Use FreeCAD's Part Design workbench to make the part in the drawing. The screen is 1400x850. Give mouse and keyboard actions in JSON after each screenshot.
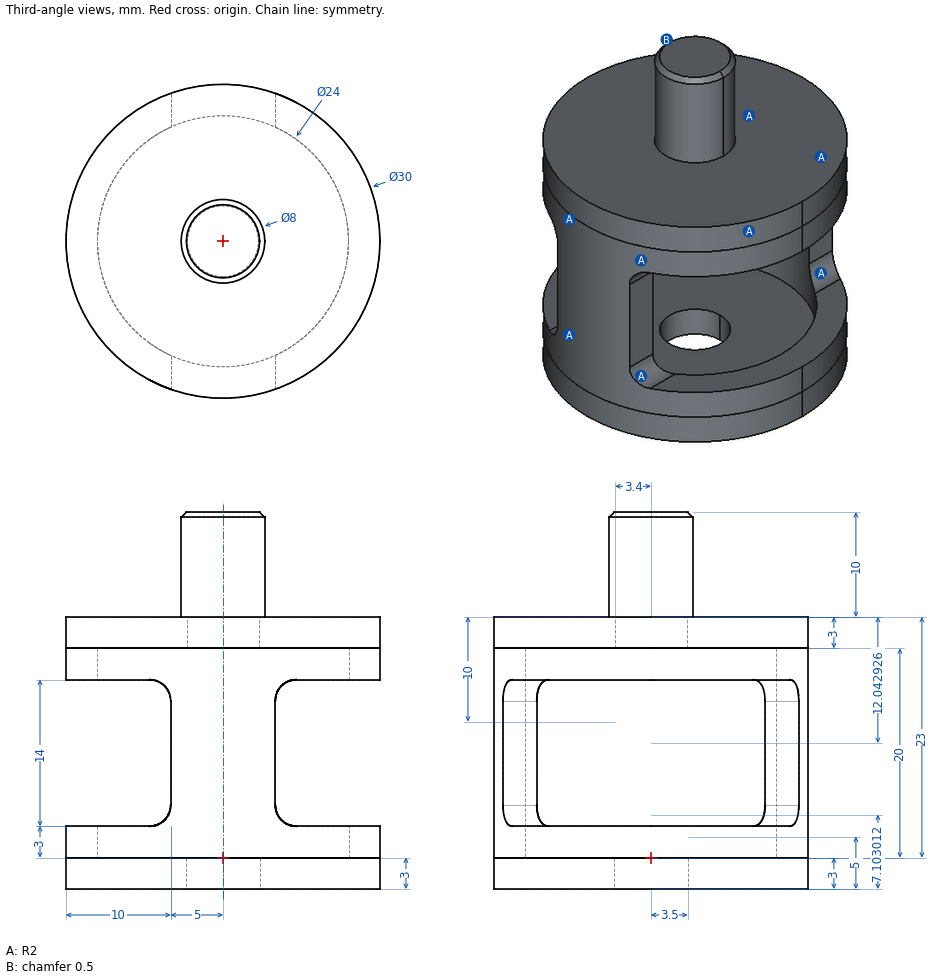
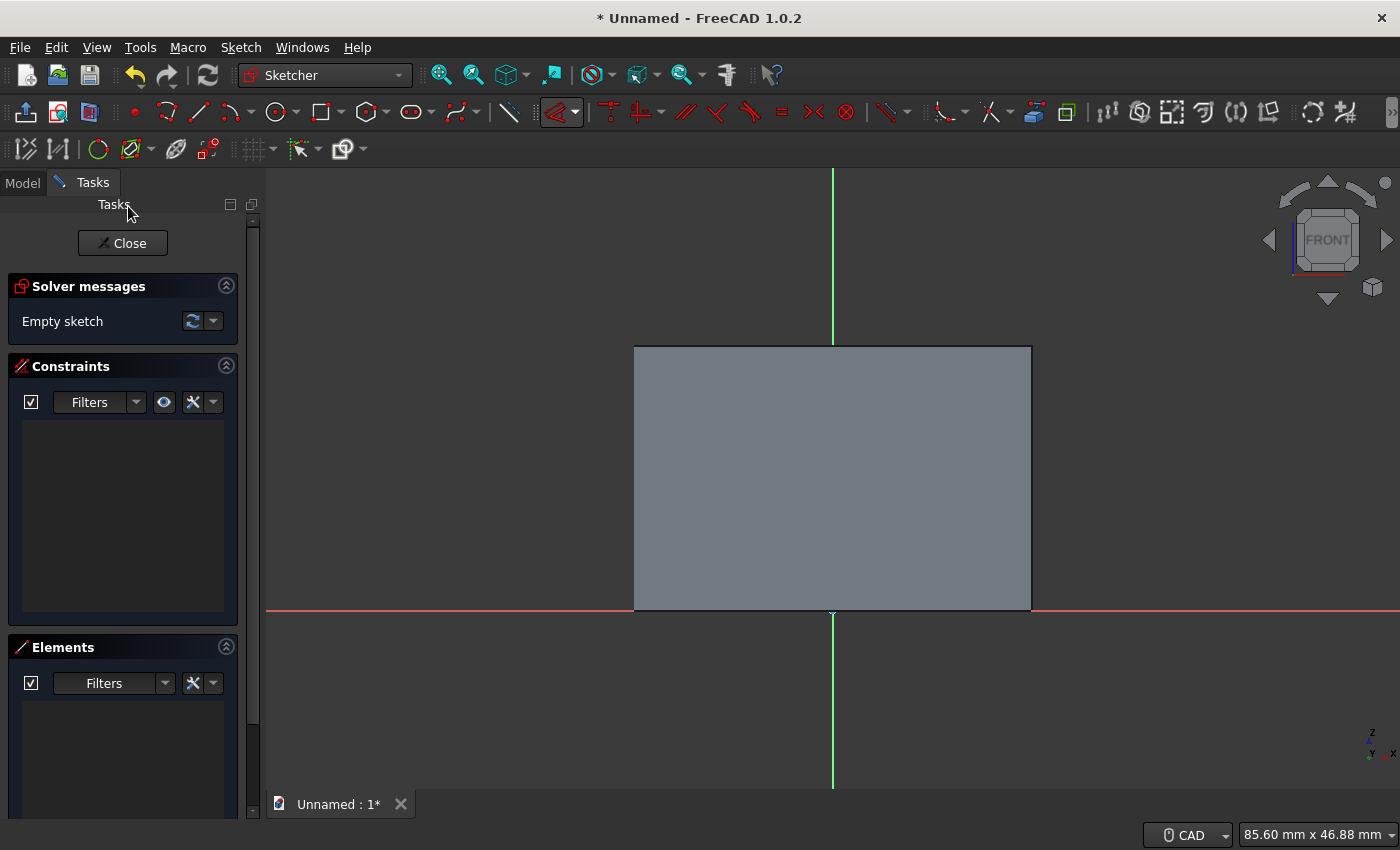
{"action": "key", "text": "q s"}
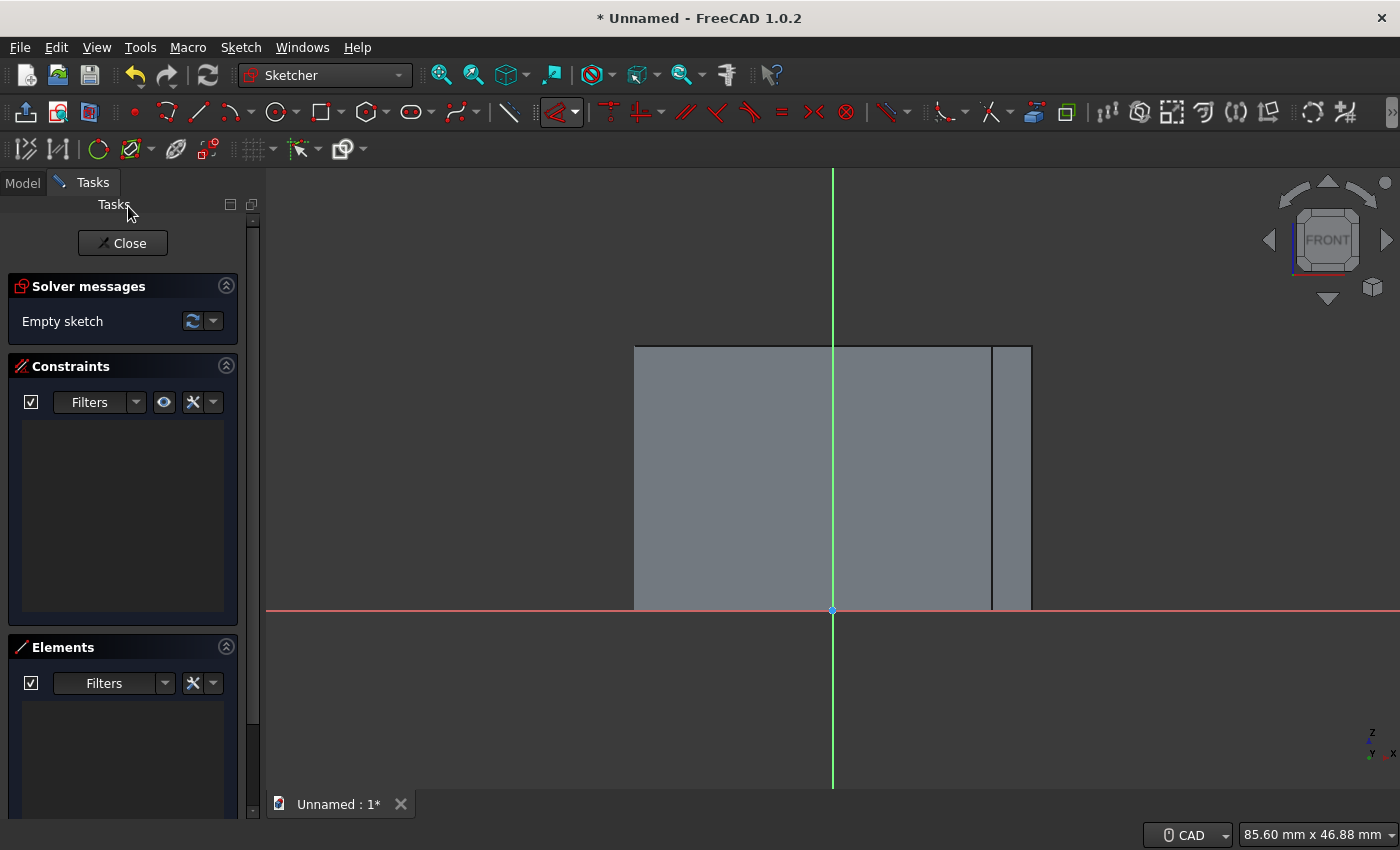
{"action": "scroll", "coordinate": [916, 523], "scroll_direction": "up", "scroll_amount": 3}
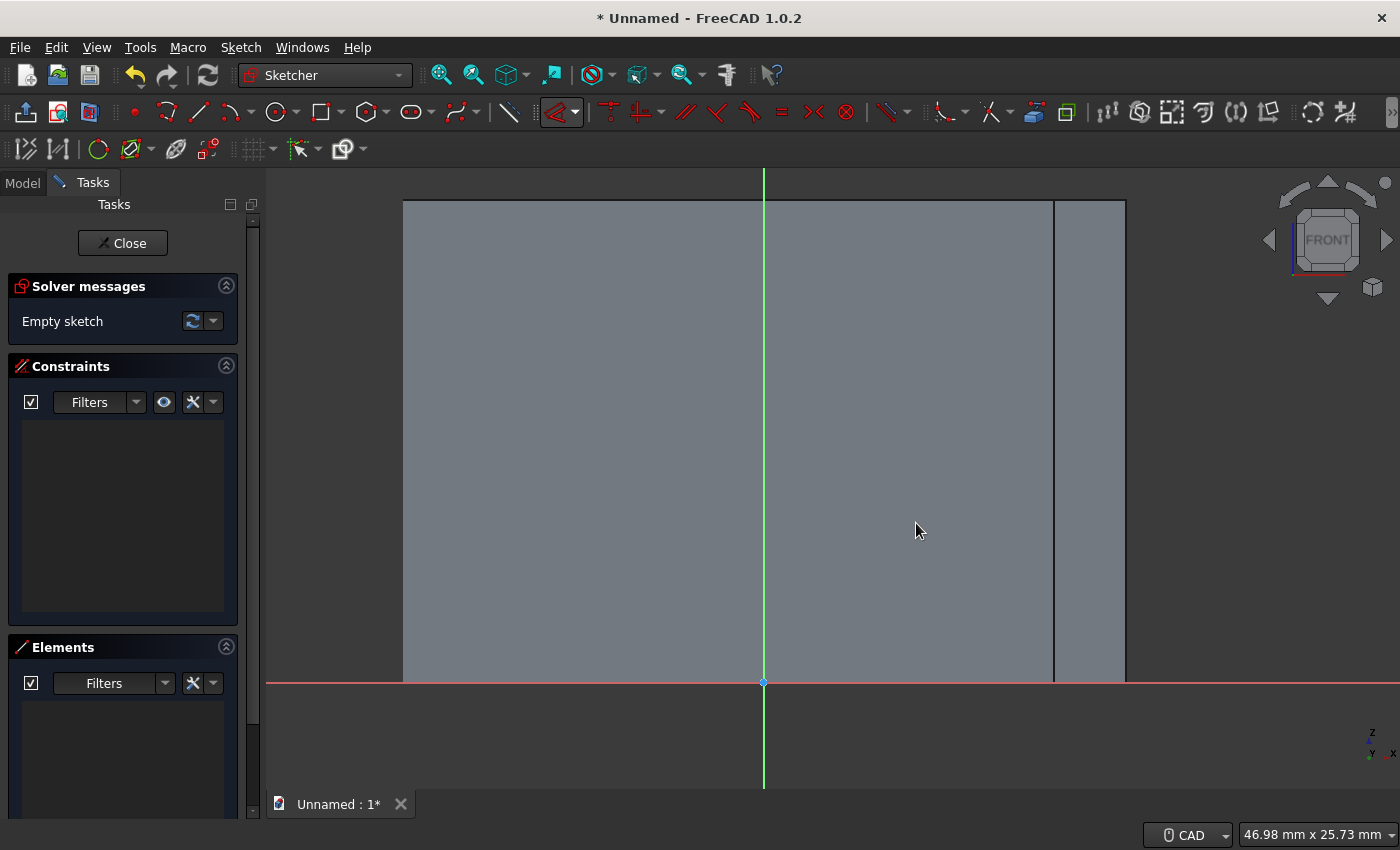
{"action": "key", "text": "g r"}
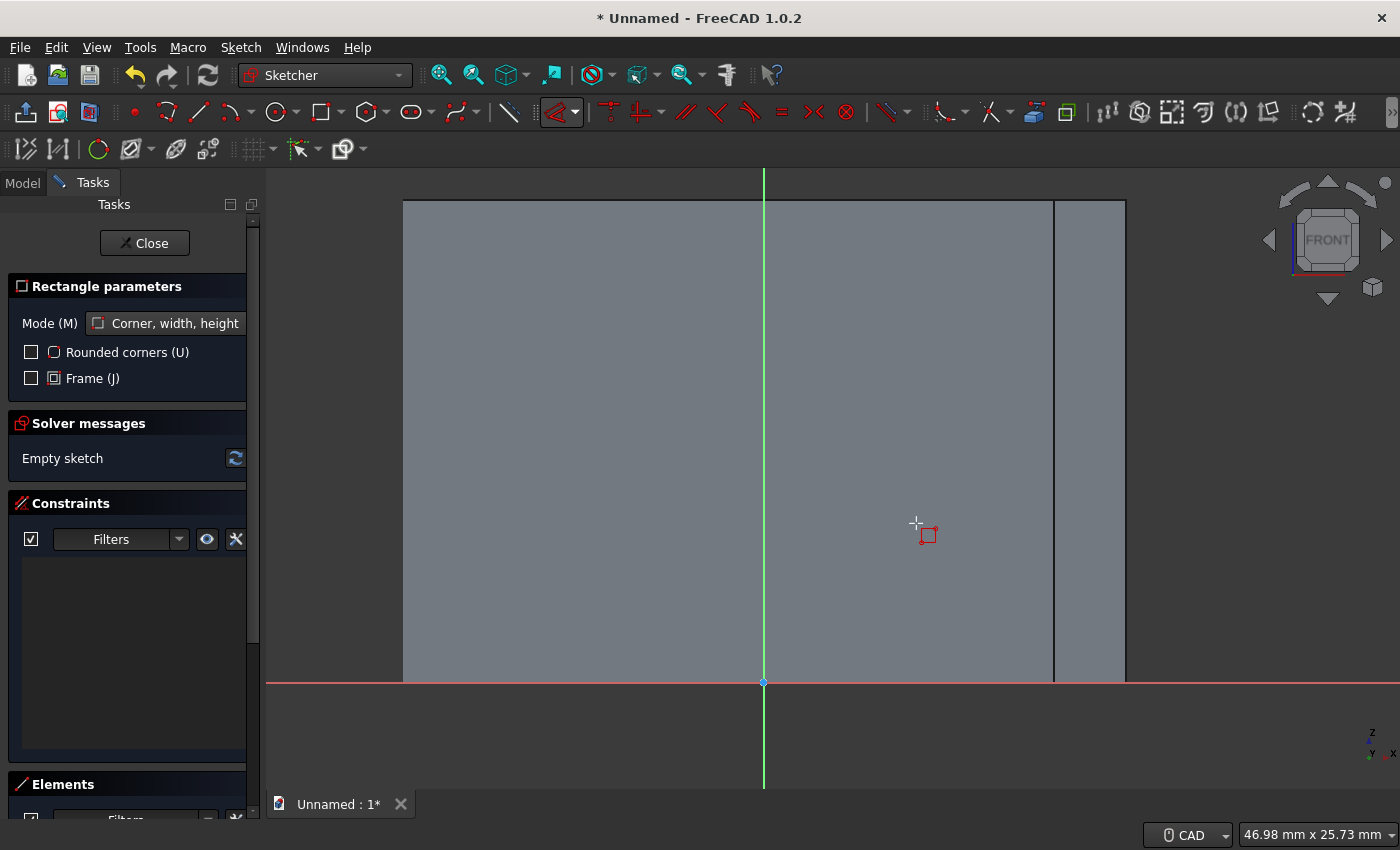
{"action": "left_click", "coordinate": [402, 272]}
{"action": "left_click", "coordinate": [643, 610]}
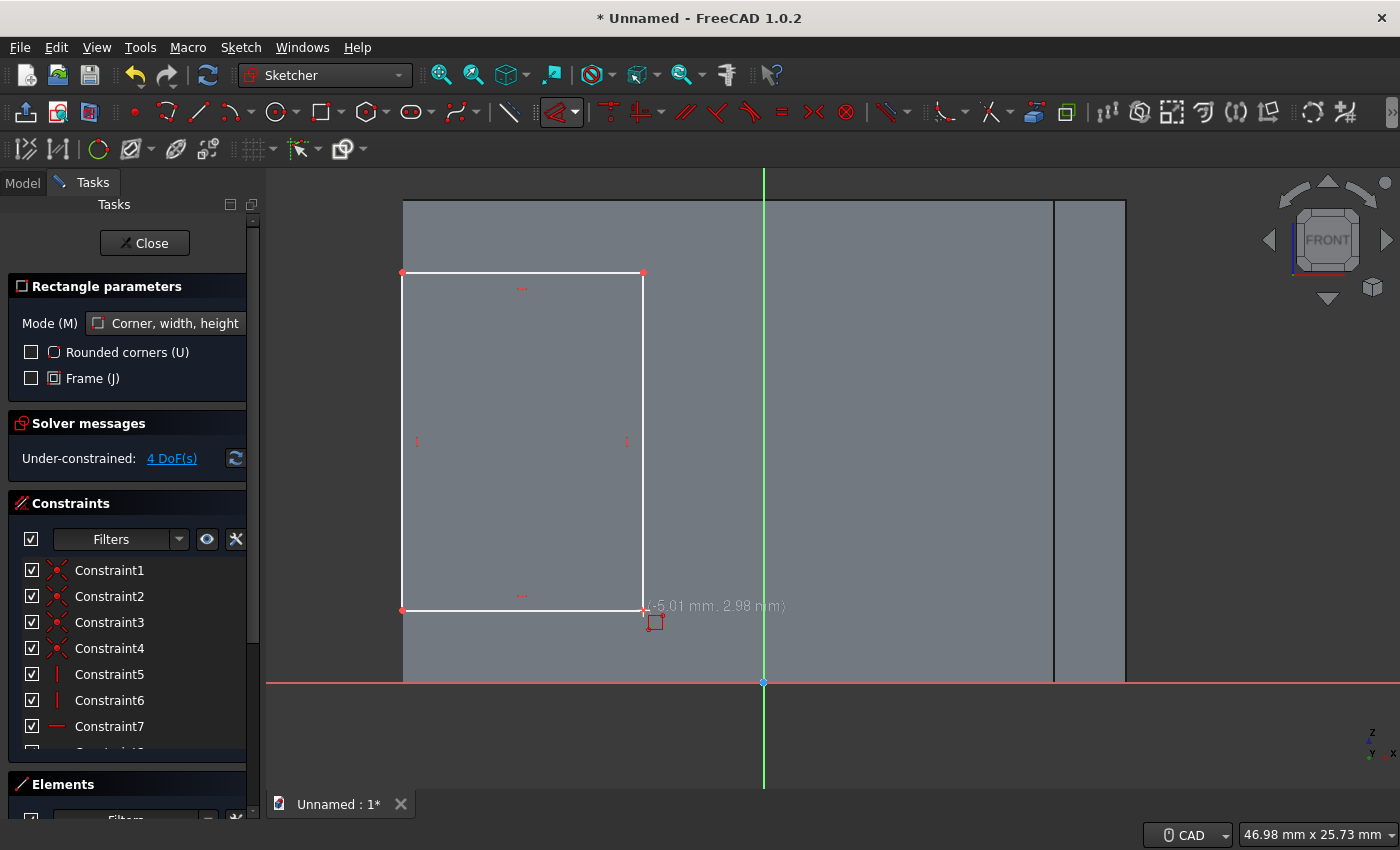
{"action": "left_click", "coordinate": [885, 272]}
{"action": "left_click", "coordinate": [1126, 610]}
{"action": "key", "text": "Escape"}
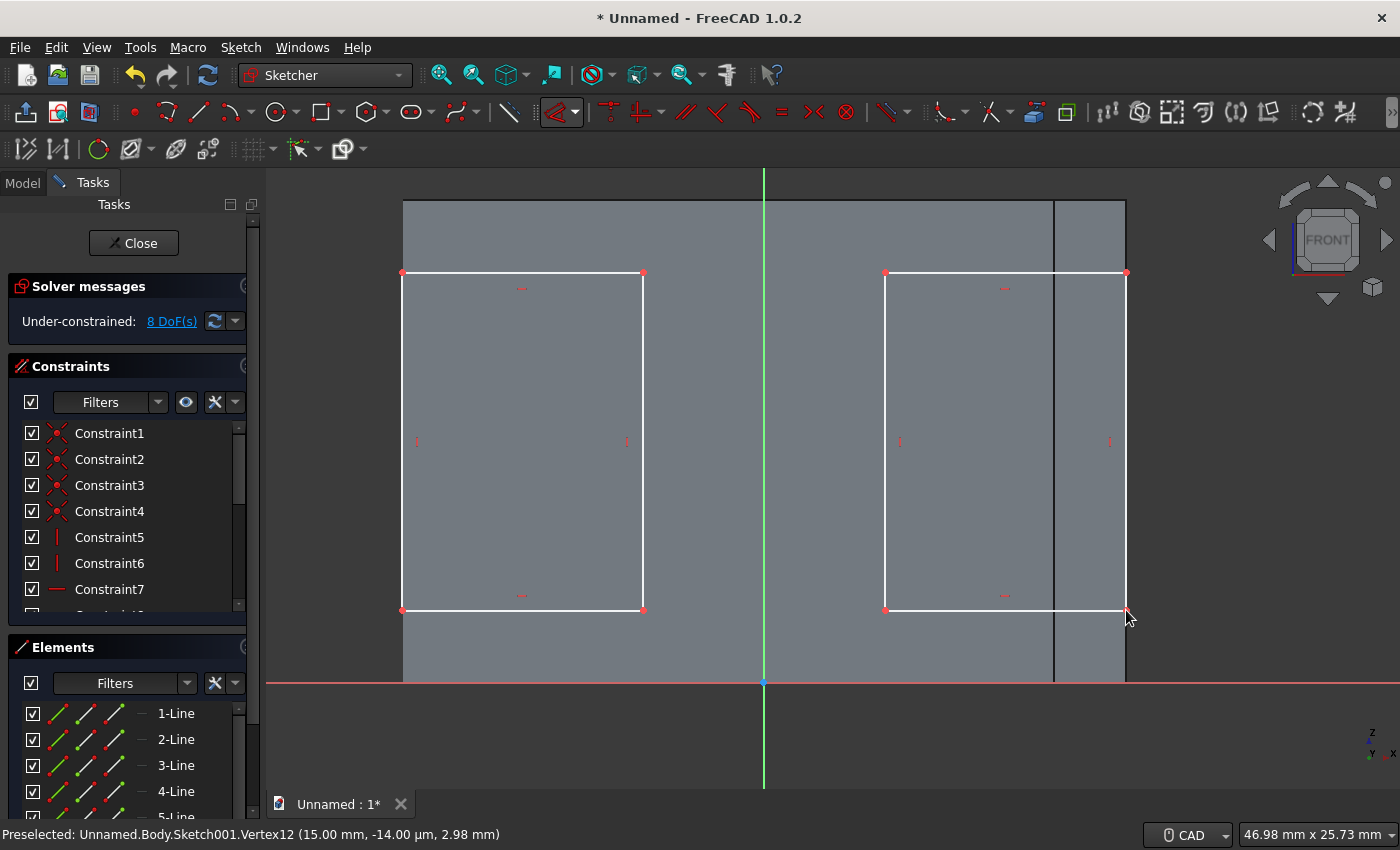
{"action": "left_click", "coordinate": [643, 273]}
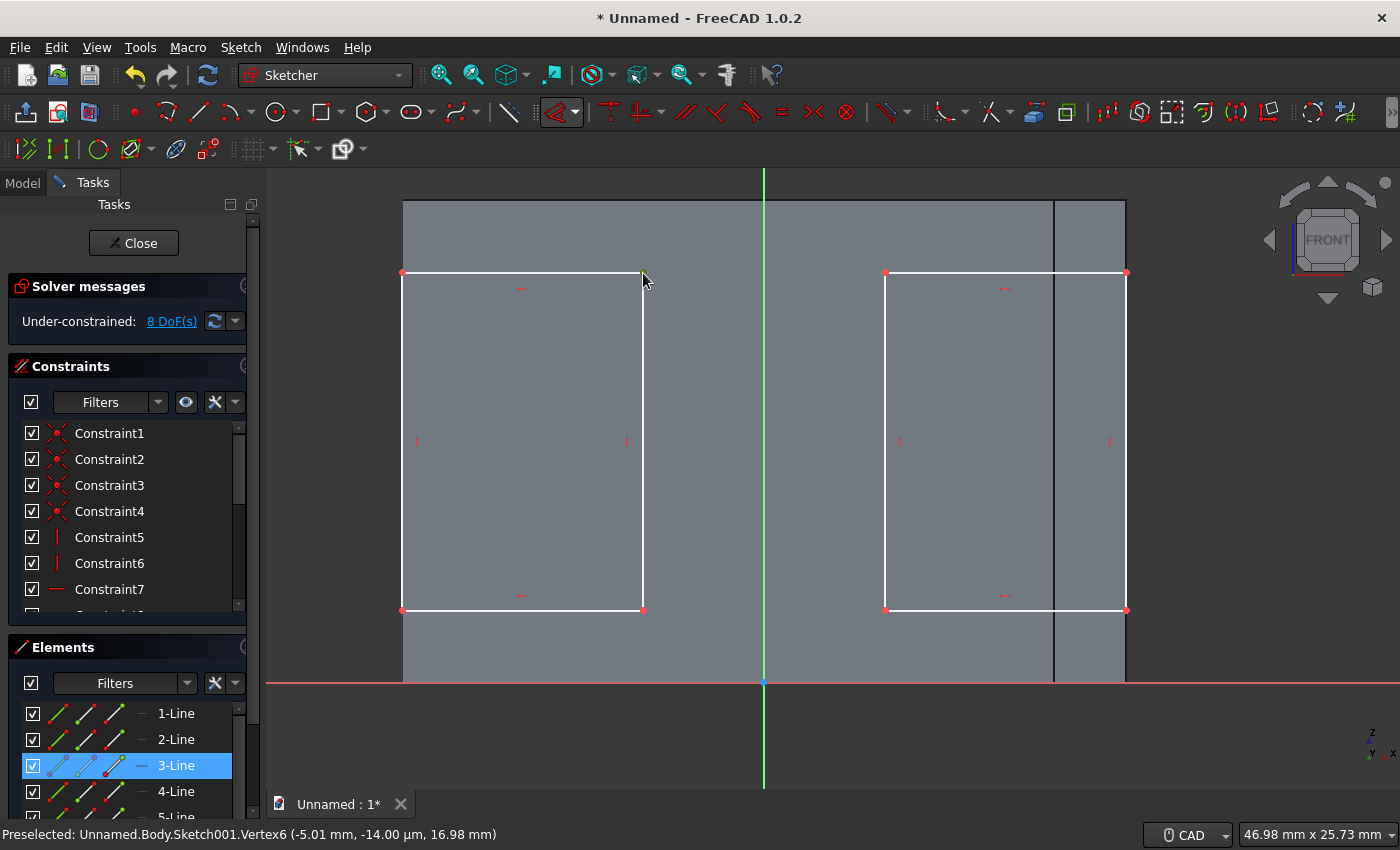
{"action": "left_click", "coordinate": [885, 273]}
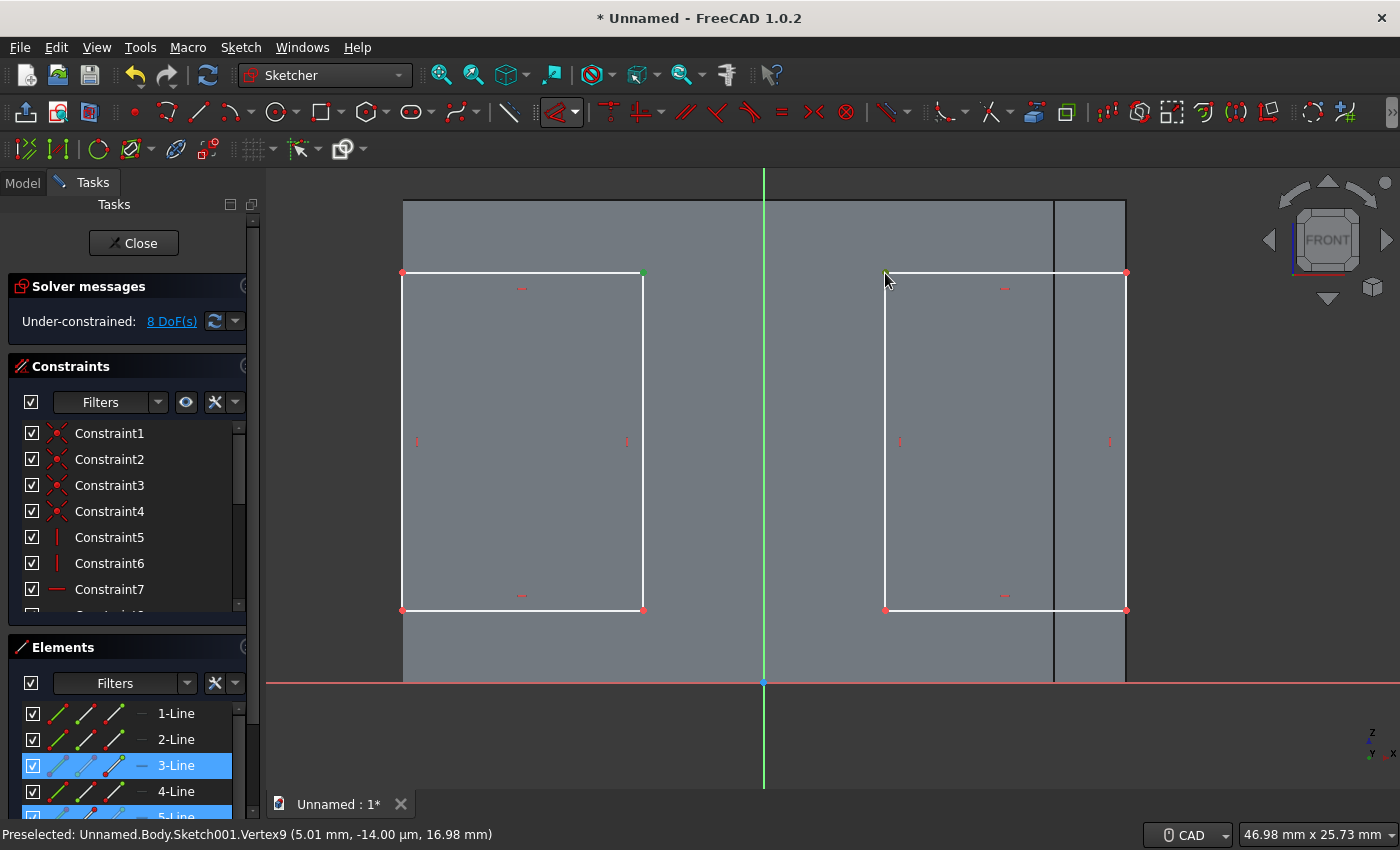
{"action": "left_click", "coordinate": [764, 721]}